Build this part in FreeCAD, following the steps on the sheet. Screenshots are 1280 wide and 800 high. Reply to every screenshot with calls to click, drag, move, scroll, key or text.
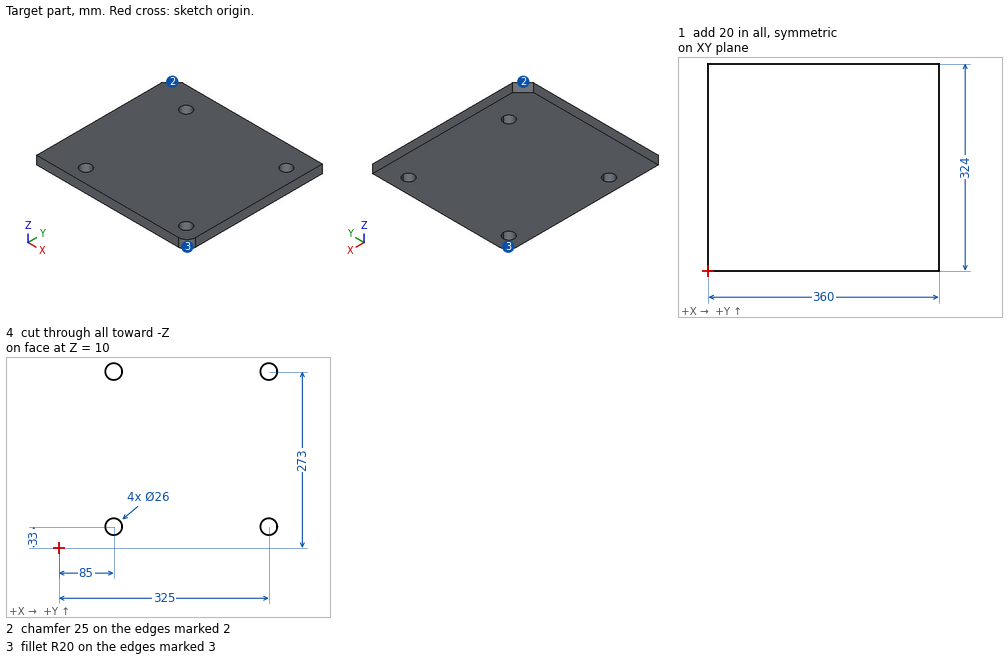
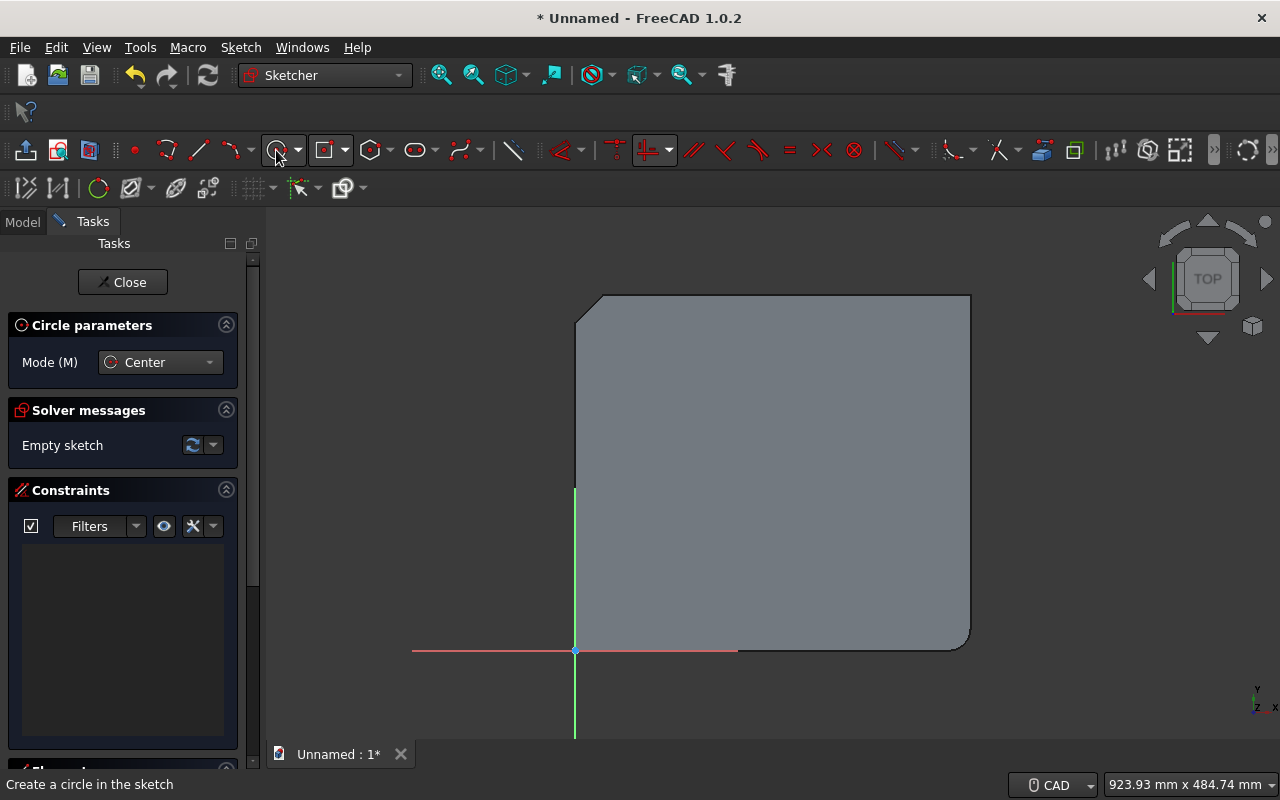
scroll(669, 615, up, 3)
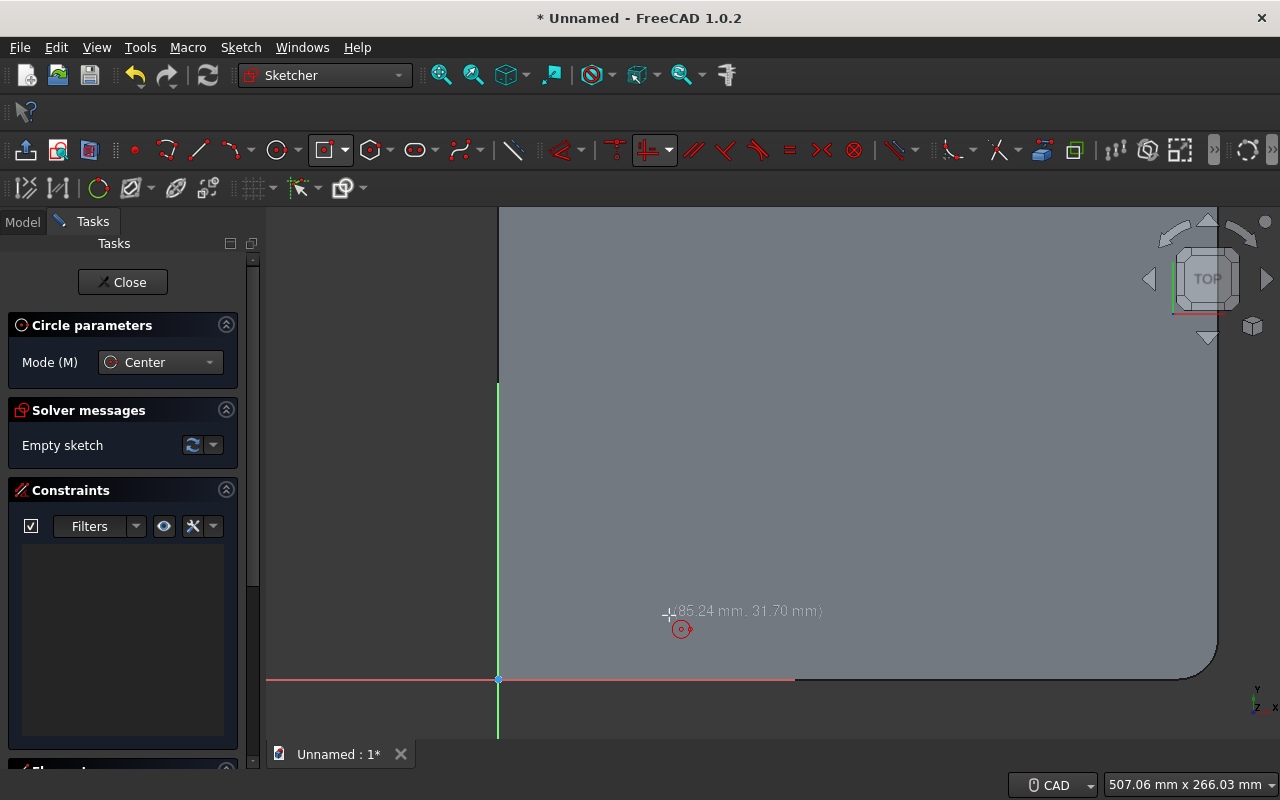
click(668, 614)
click(687, 595)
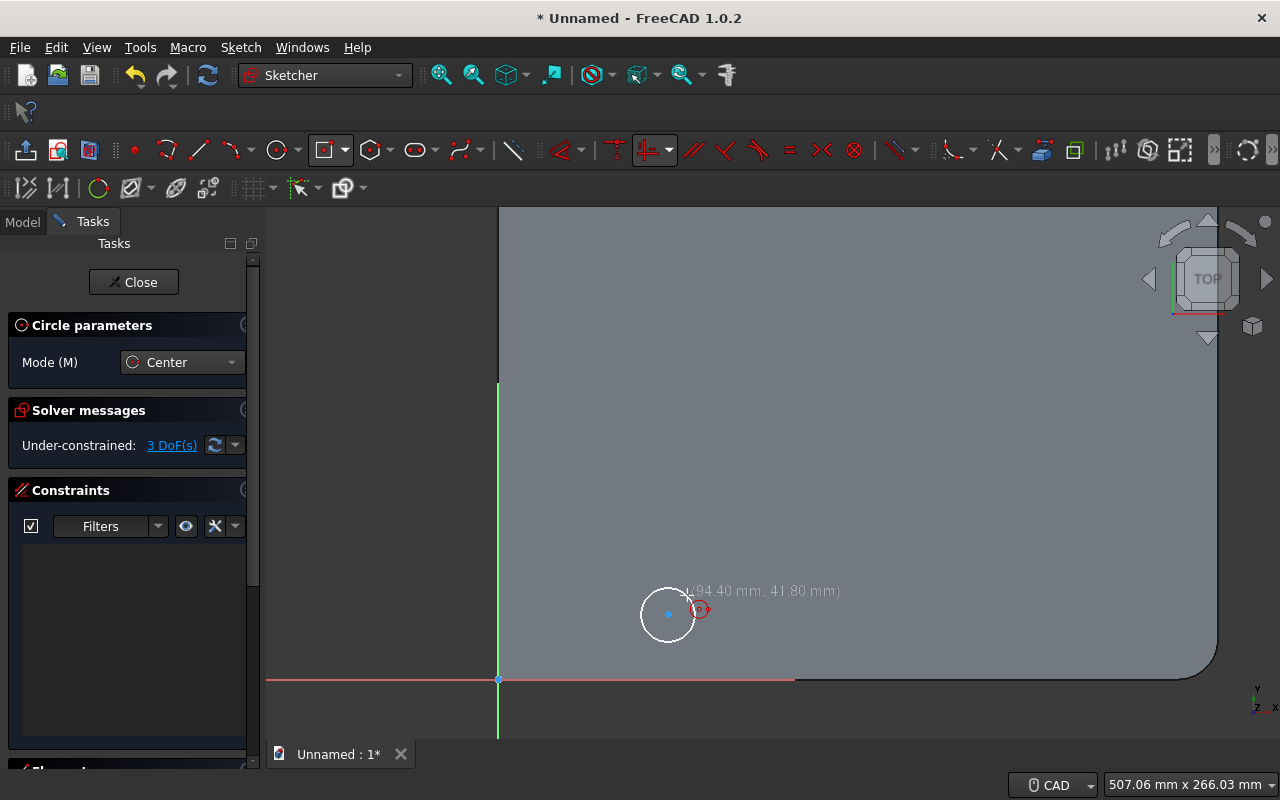
scroll(544, 570, down, 3)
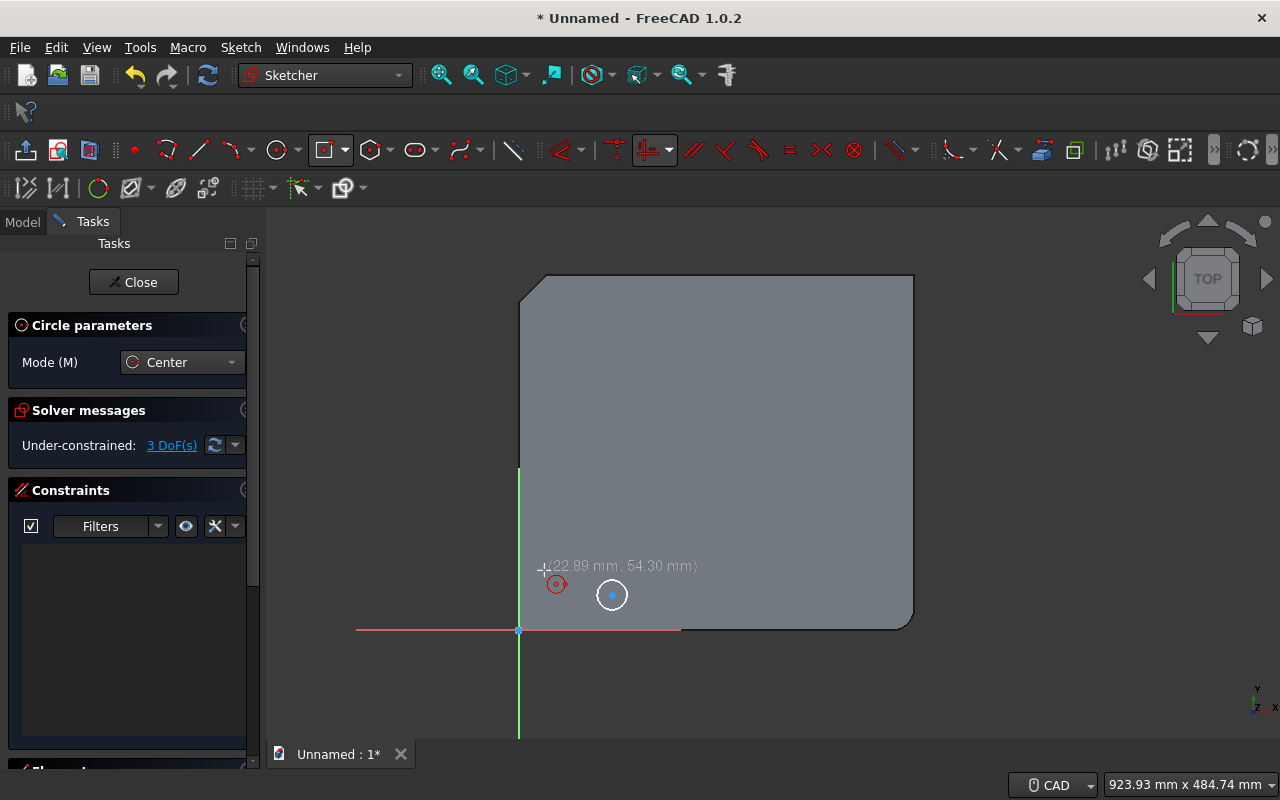
scroll(876, 594, up, 3)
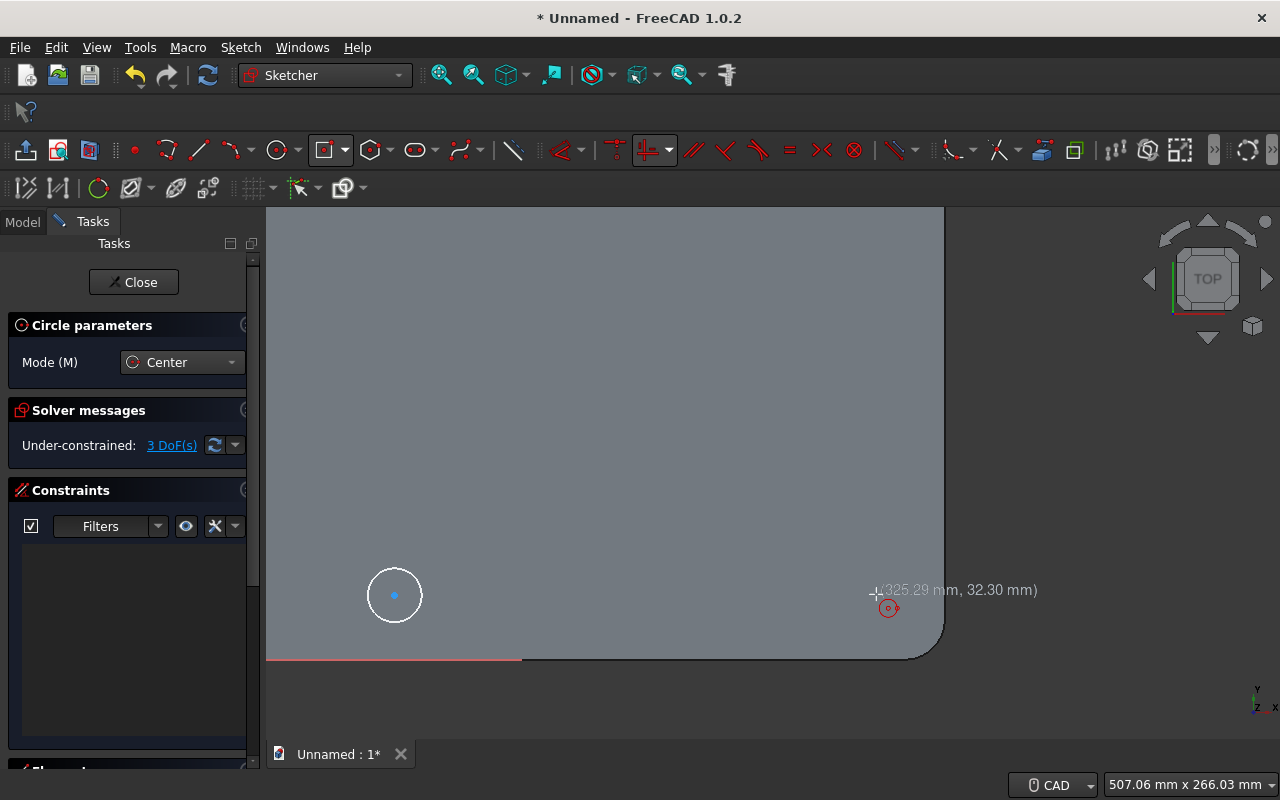
click(875, 594)
click(893, 575)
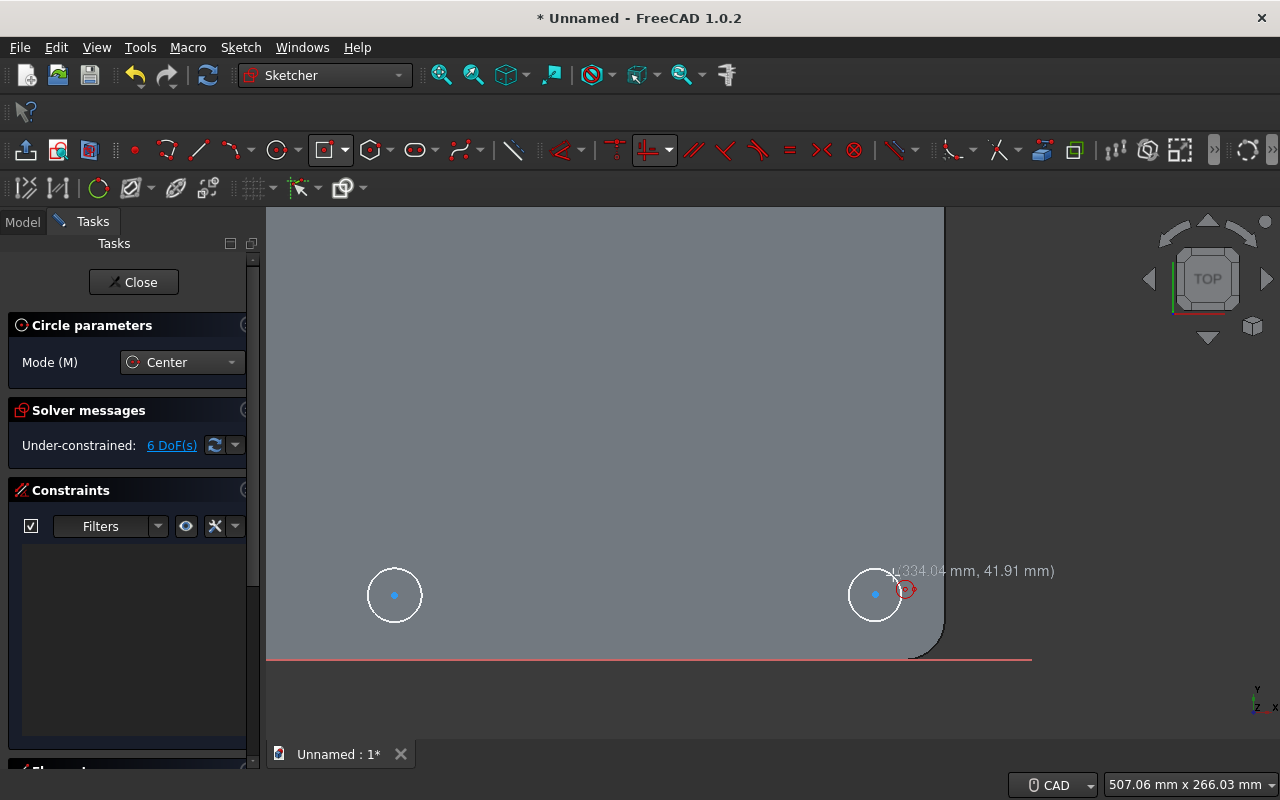
scroll(877, 594, down, 3)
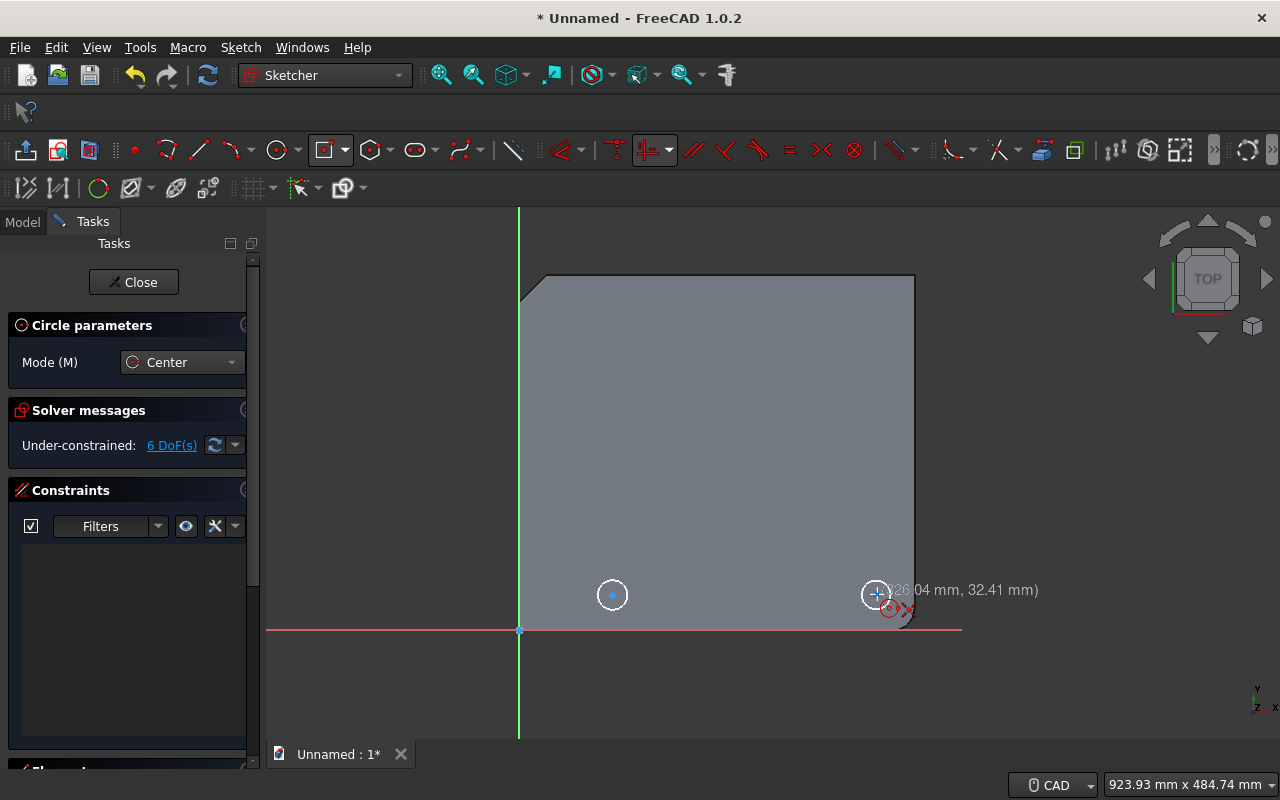
scroll(876, 331, up, 3)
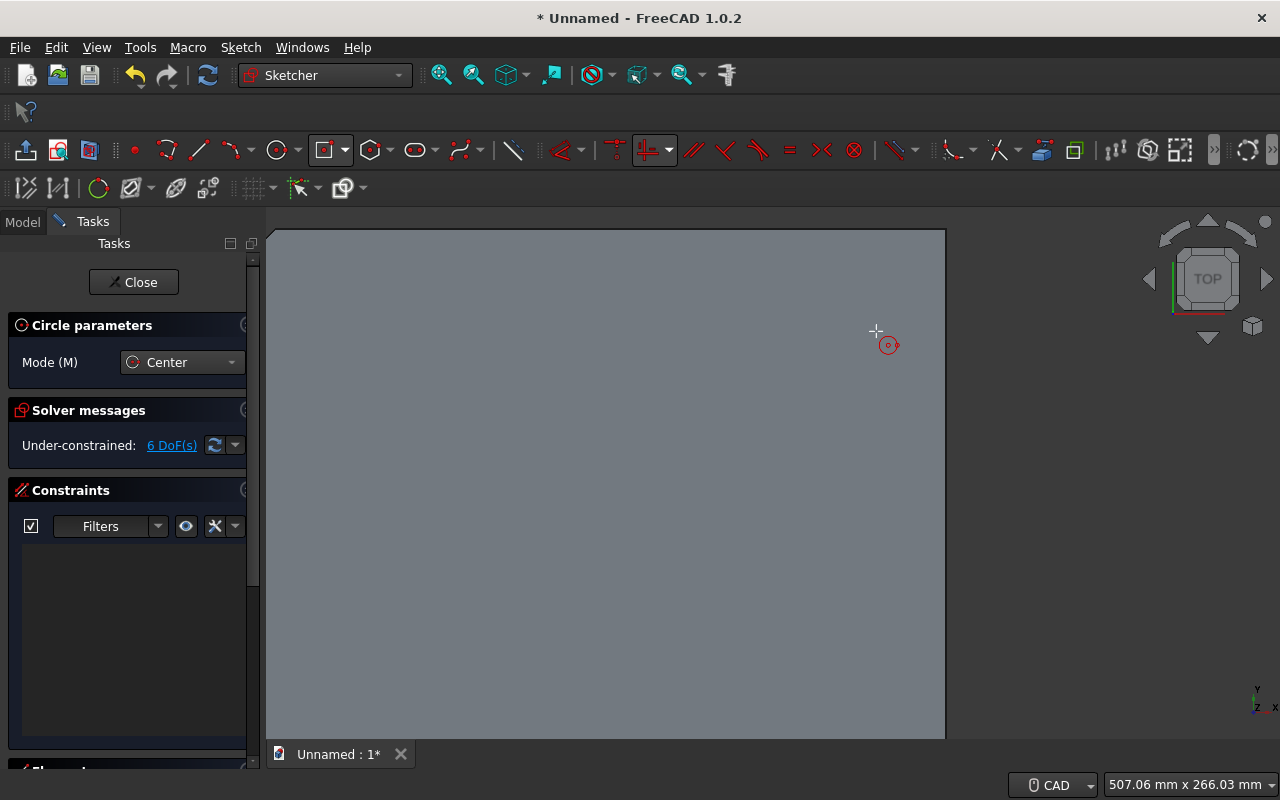
click(876, 331)
click(894, 312)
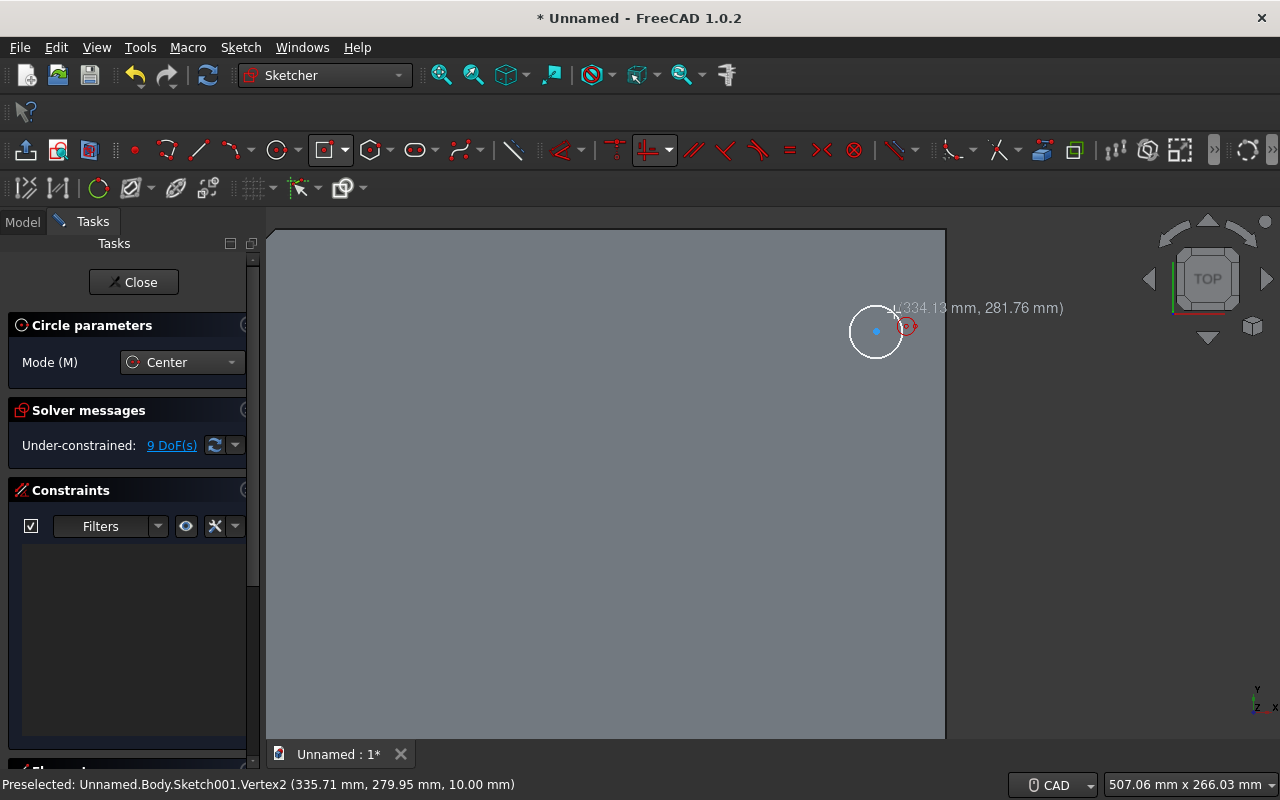
click(396, 331)
click(414, 312)
key(Escape)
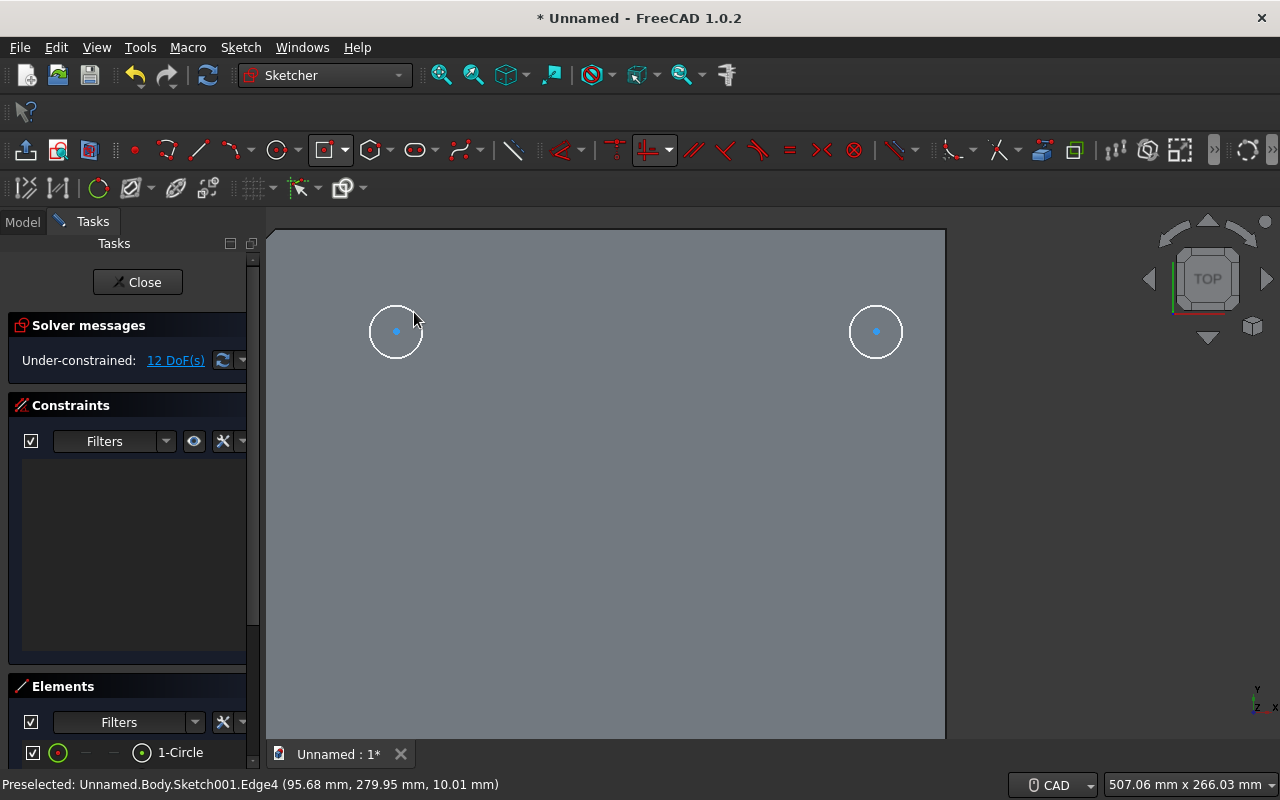
scroll(876, 330, down, 3)